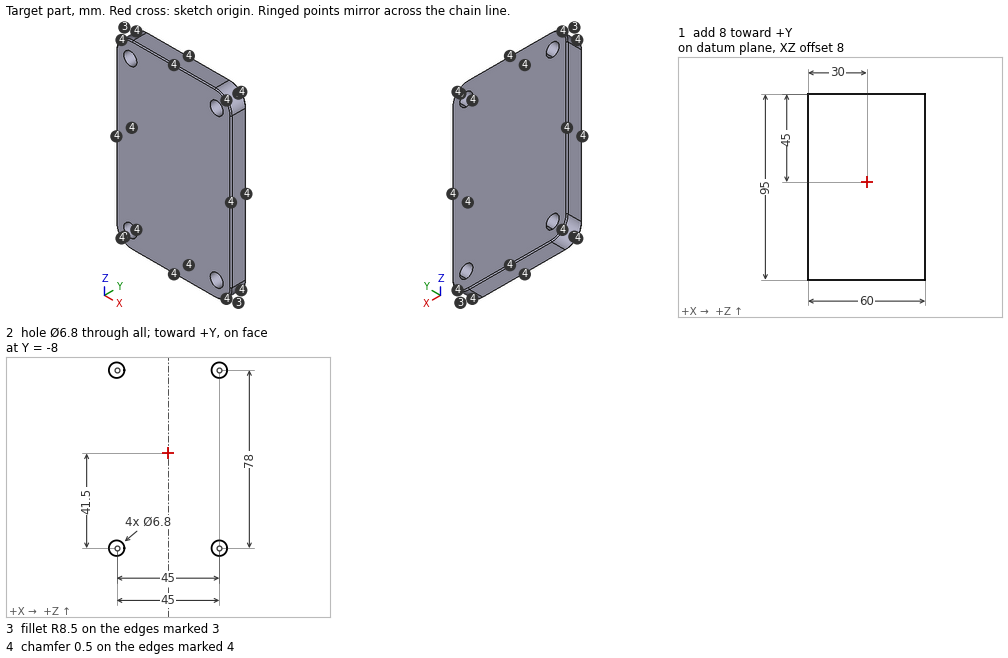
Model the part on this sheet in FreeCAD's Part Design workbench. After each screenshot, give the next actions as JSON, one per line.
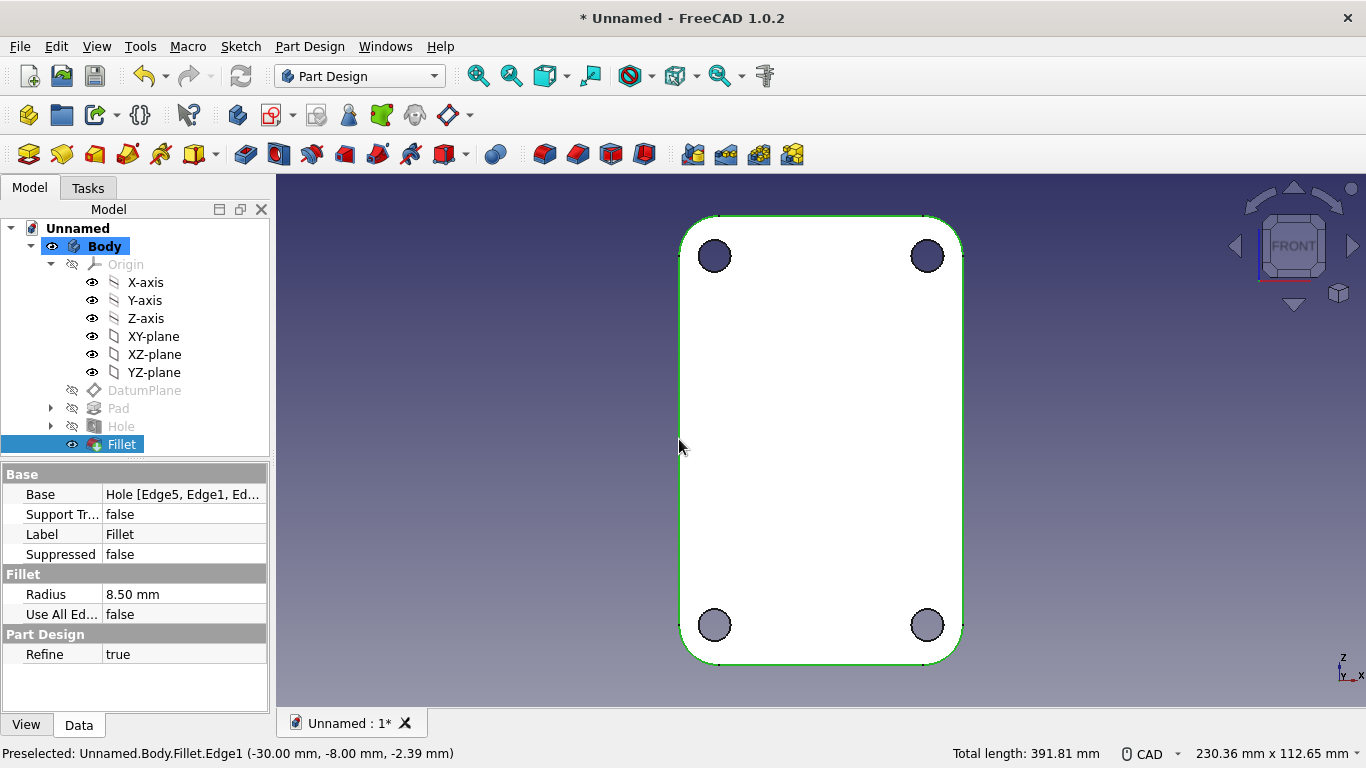
{"action": "key", "text": "3"}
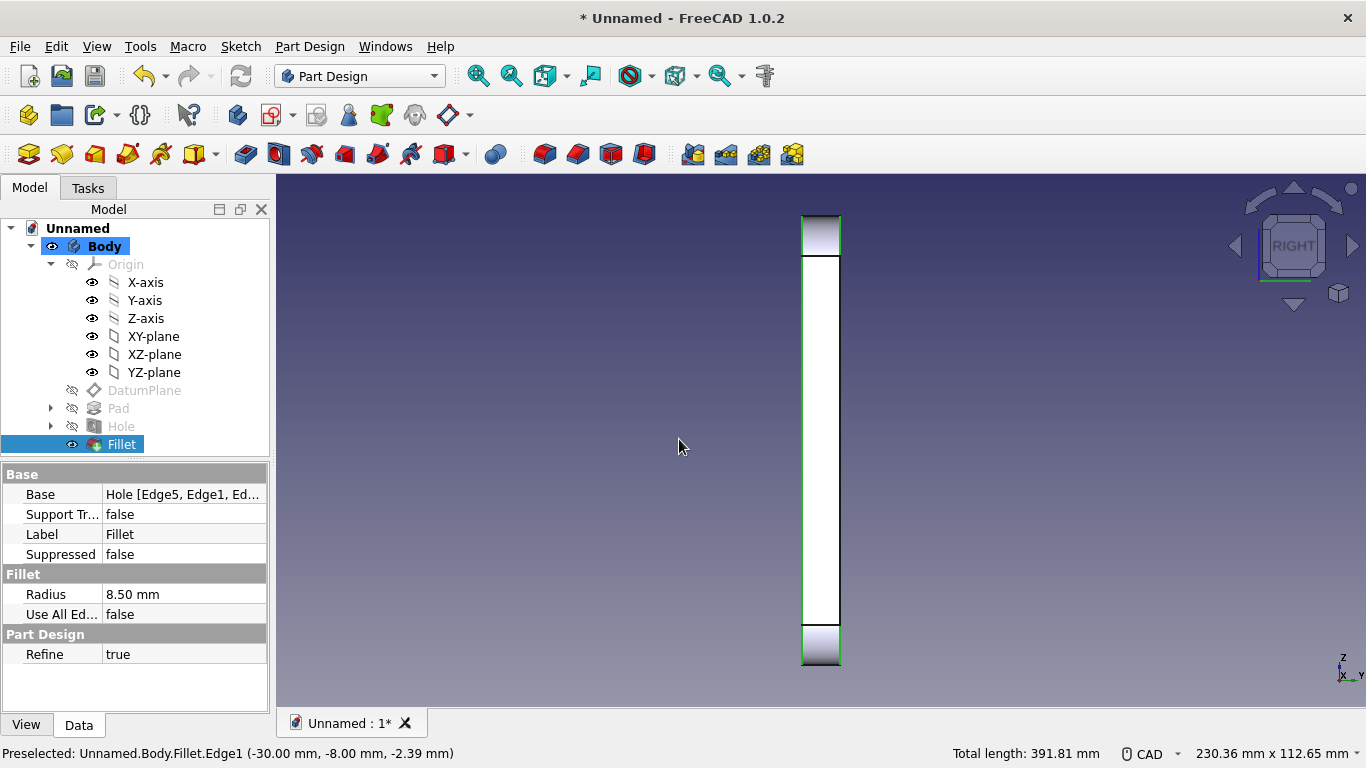
{"action": "left_click", "coordinate": [840, 439], "text": "ctrl"}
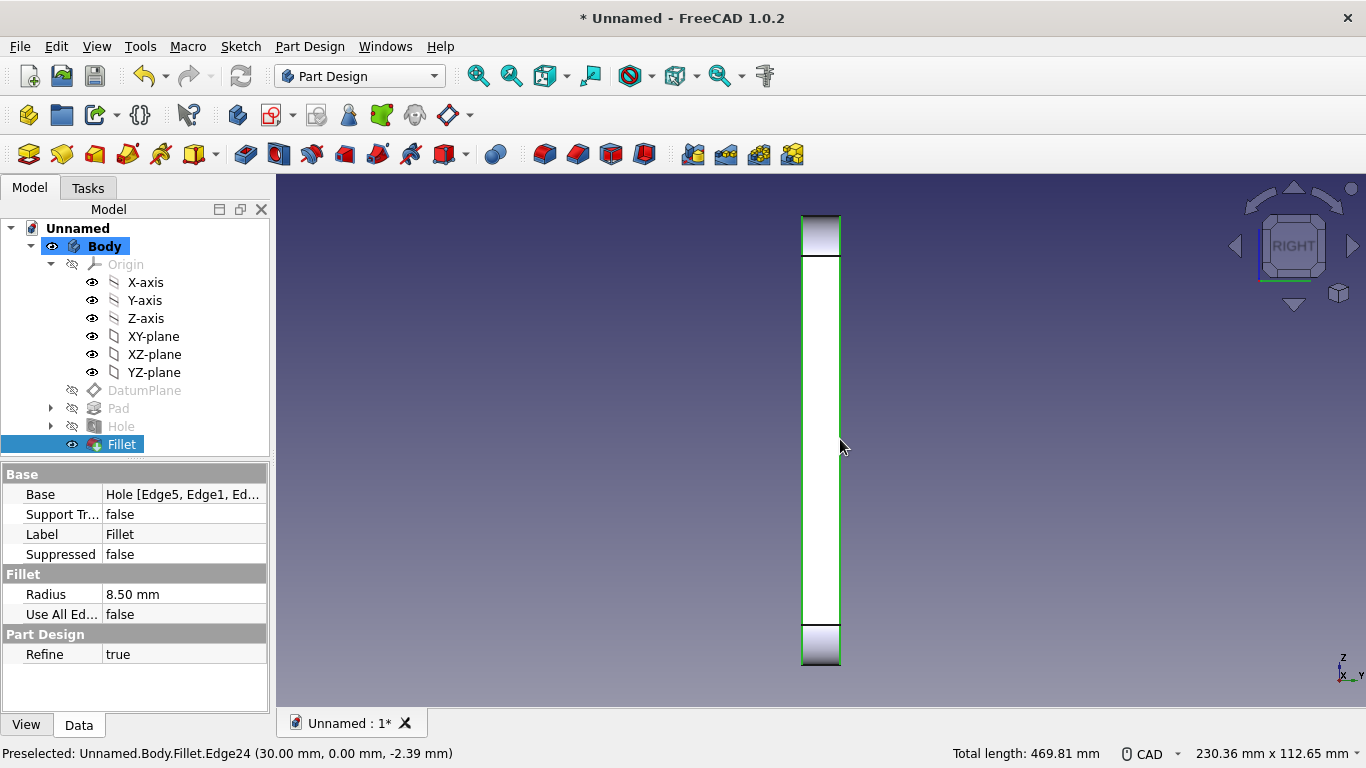
{"action": "key", "text": "5"}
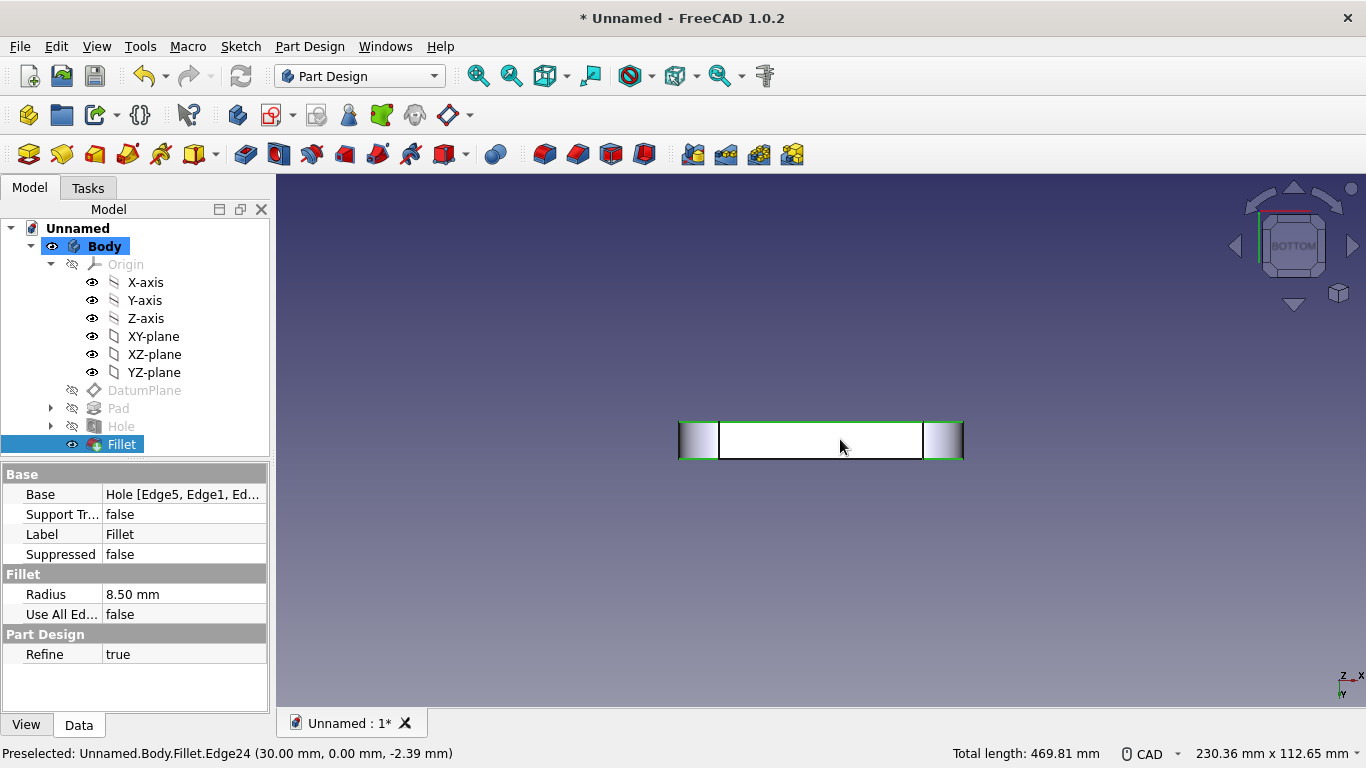
{"action": "left_click", "coordinate": [479, 76]}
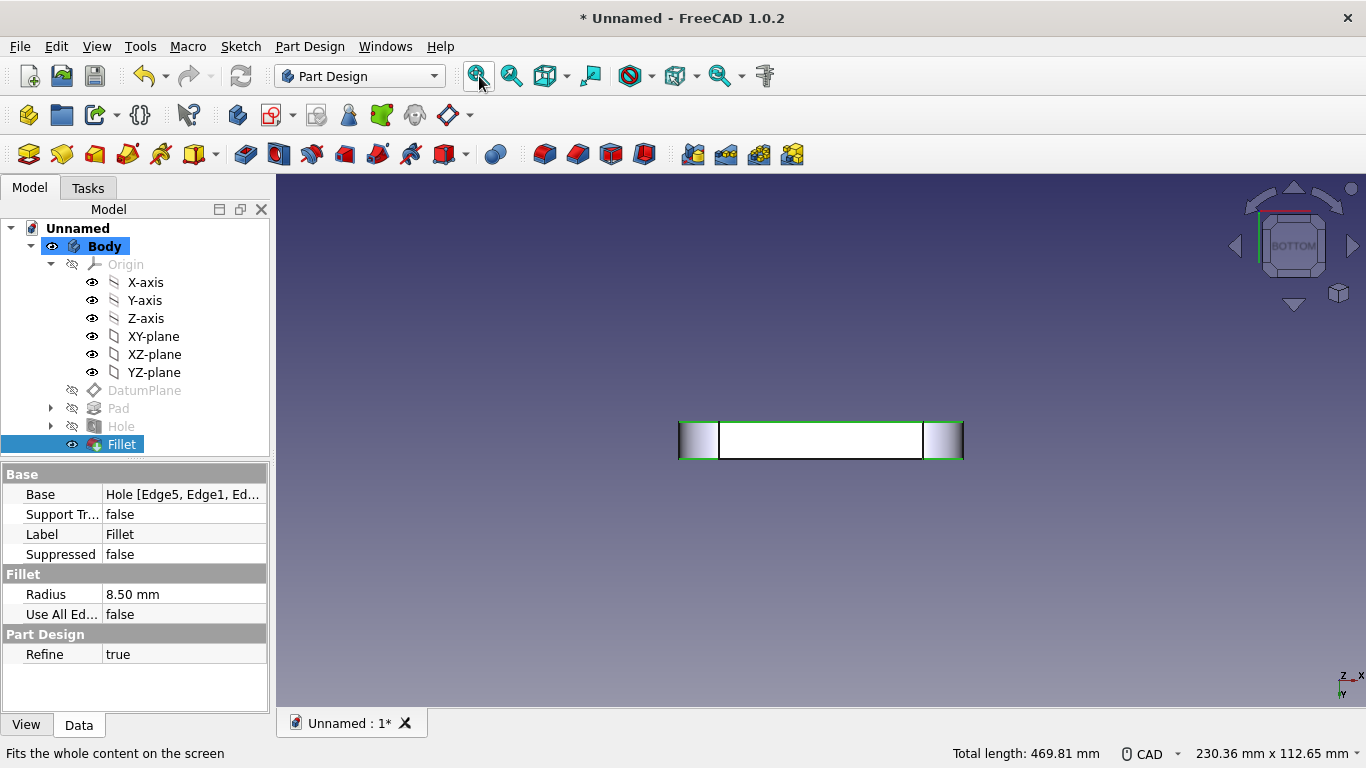
{"action": "key", "text": "4"}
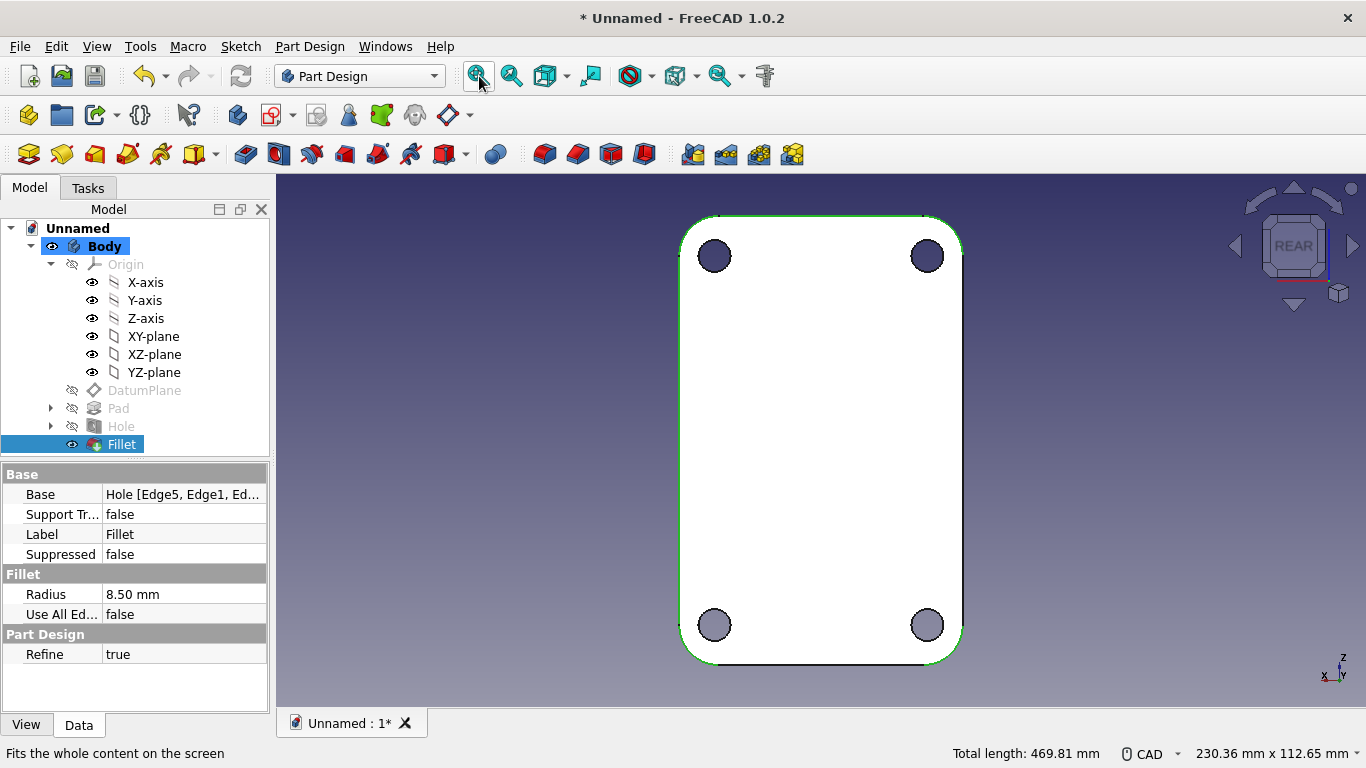
{"action": "left_click", "coordinate": [821, 664], "text": "ctrl"}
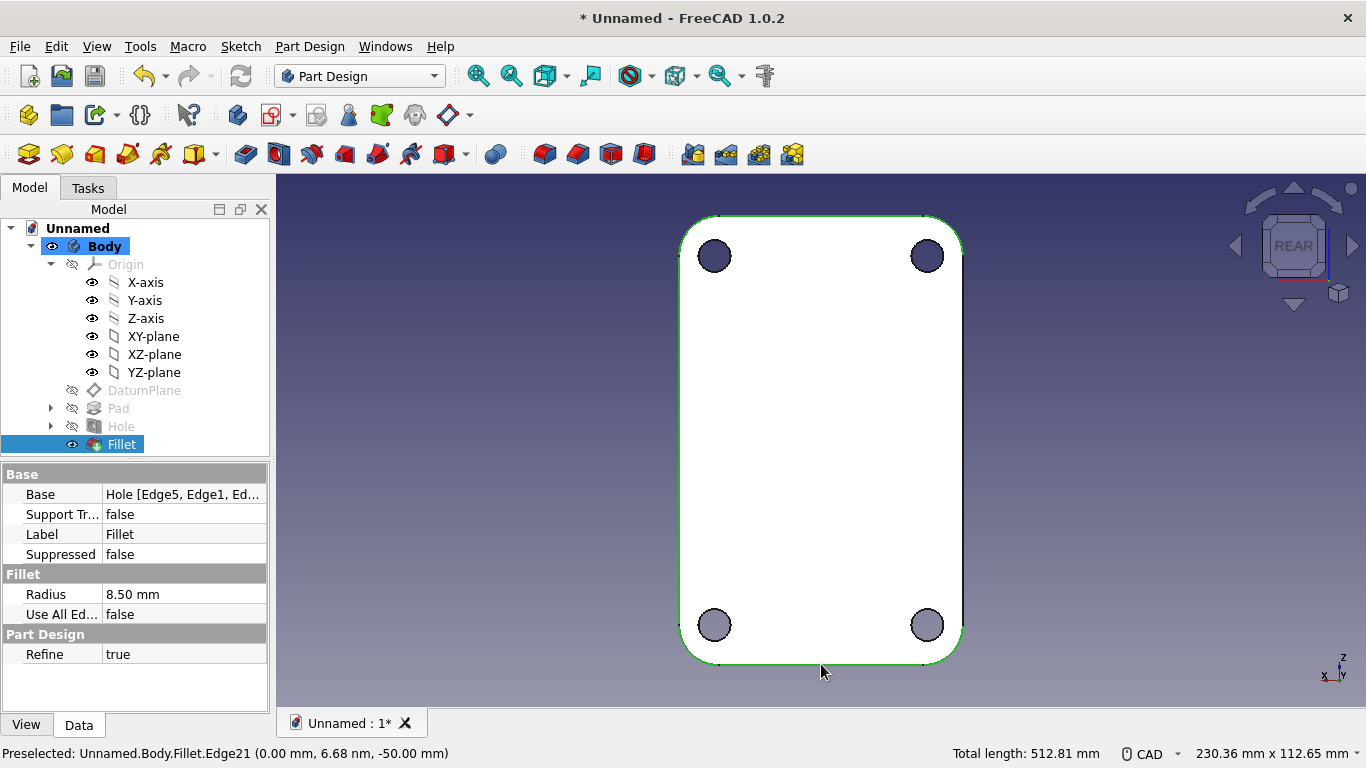
{"action": "left_click", "coordinate": [963, 439], "text": "ctrl"}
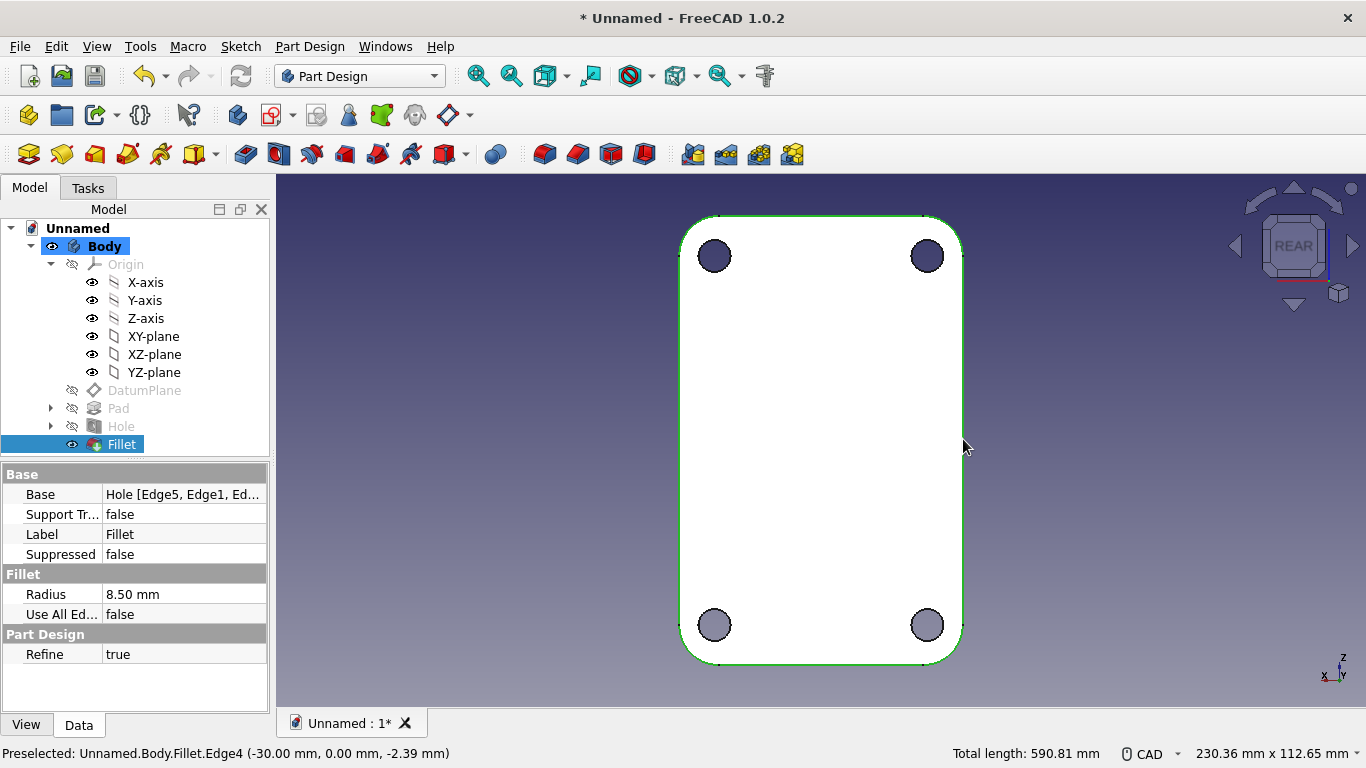
{"action": "left_click", "coordinate": [578, 154]}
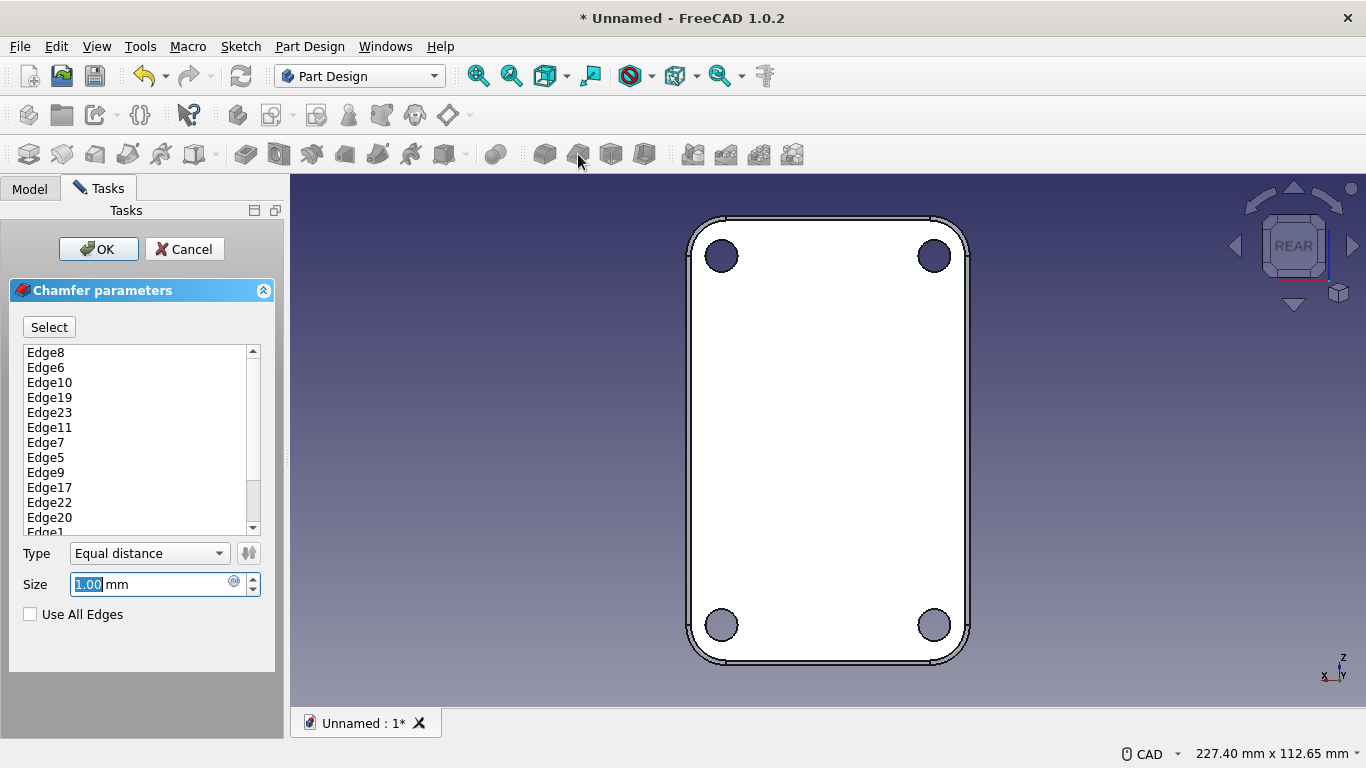
{"action": "type", "text": "0.5"}
{"action": "key", "text": "Tab"}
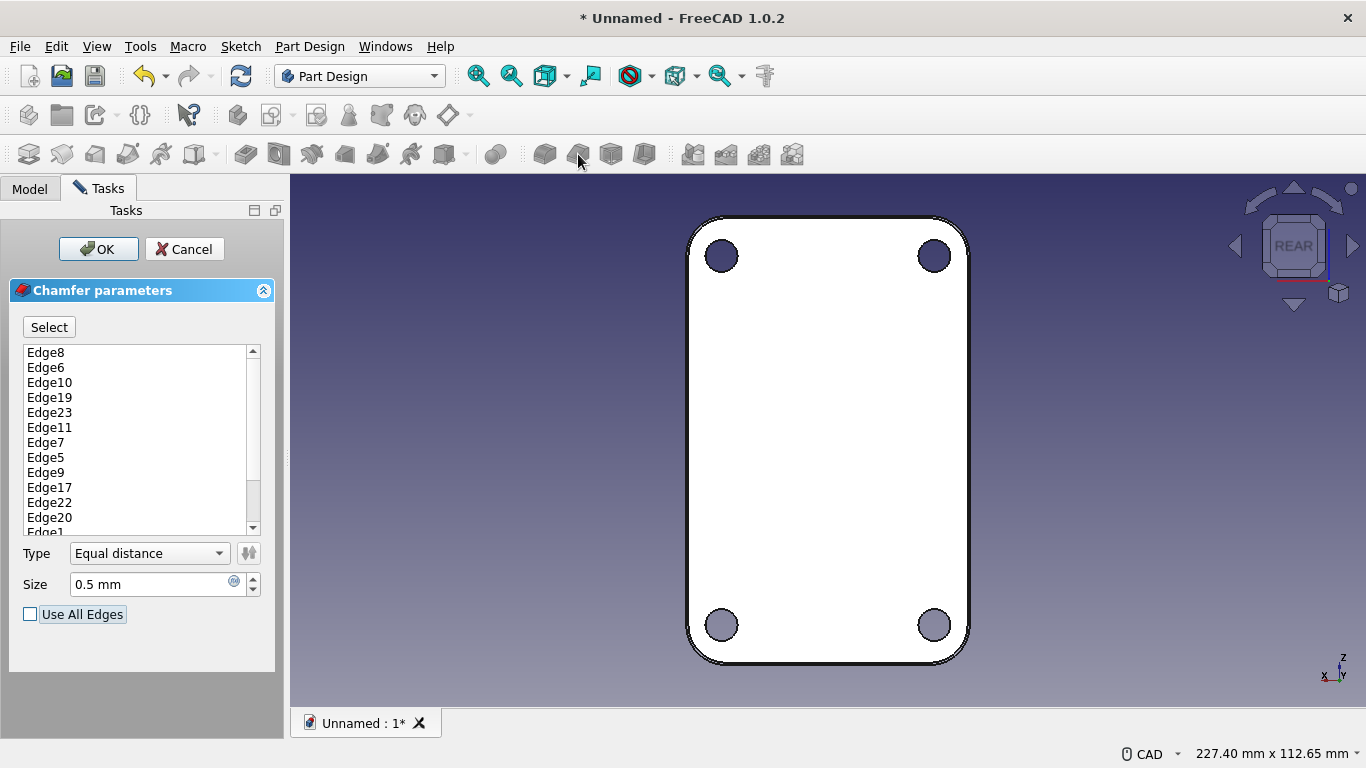
{"action": "left_click", "coordinate": [99, 249]}